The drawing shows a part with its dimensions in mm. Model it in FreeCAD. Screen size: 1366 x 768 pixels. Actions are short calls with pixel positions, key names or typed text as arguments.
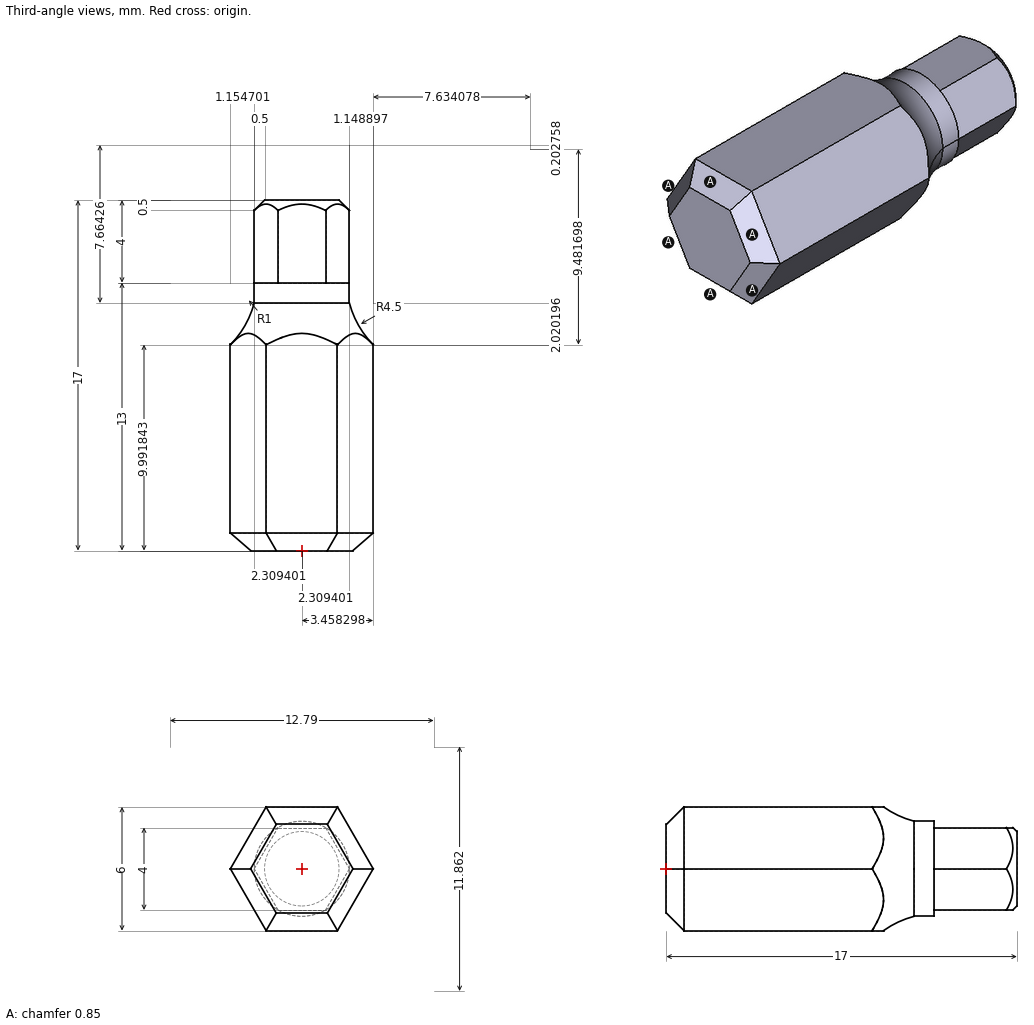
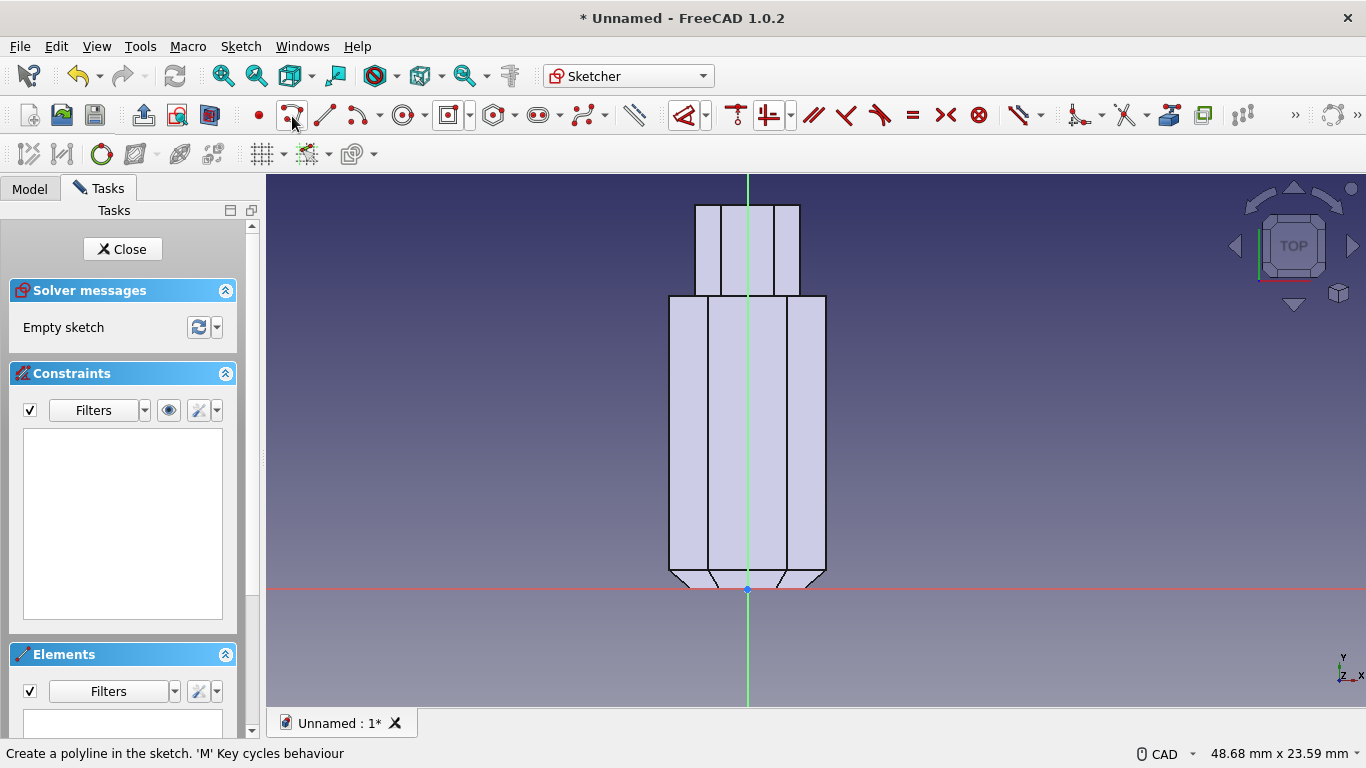
click(695, 296)
click(669, 296)
click(669, 318)
right_click(669, 318)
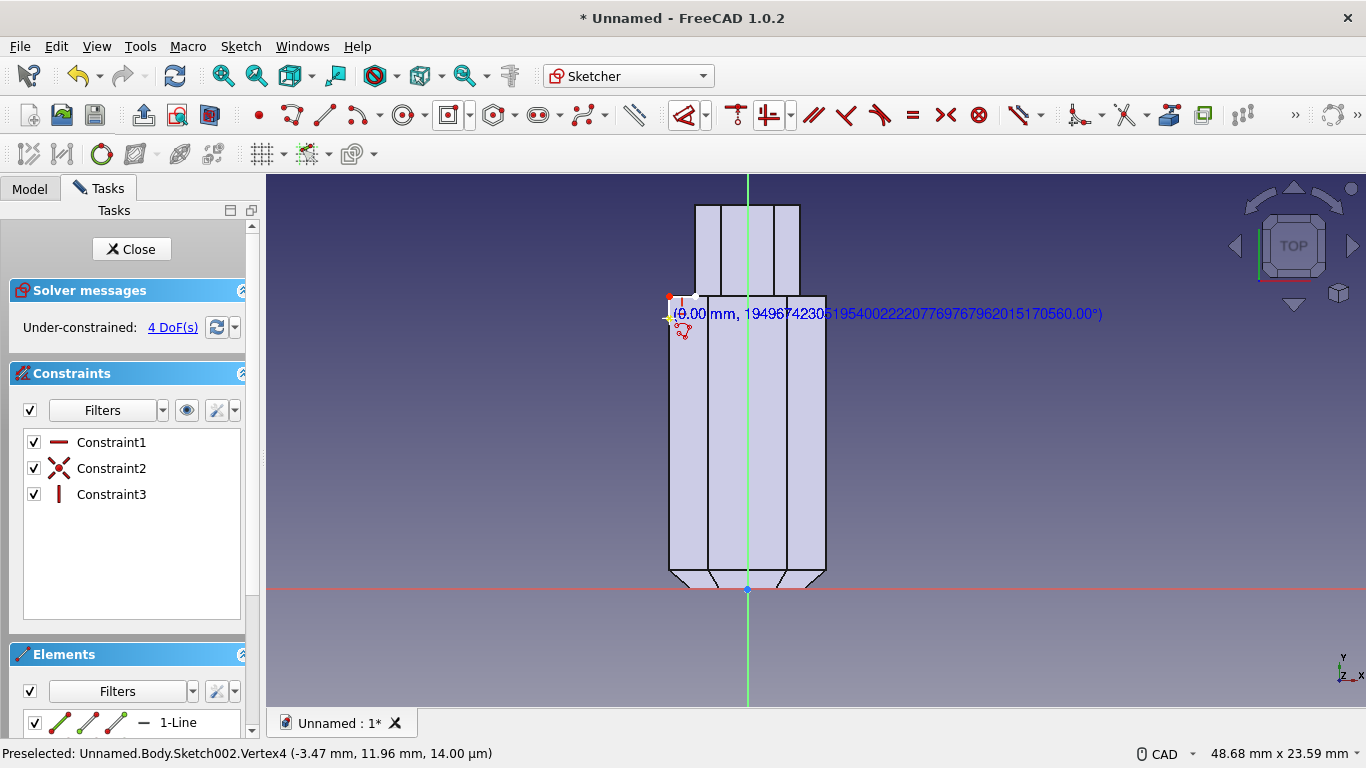
click(380, 116)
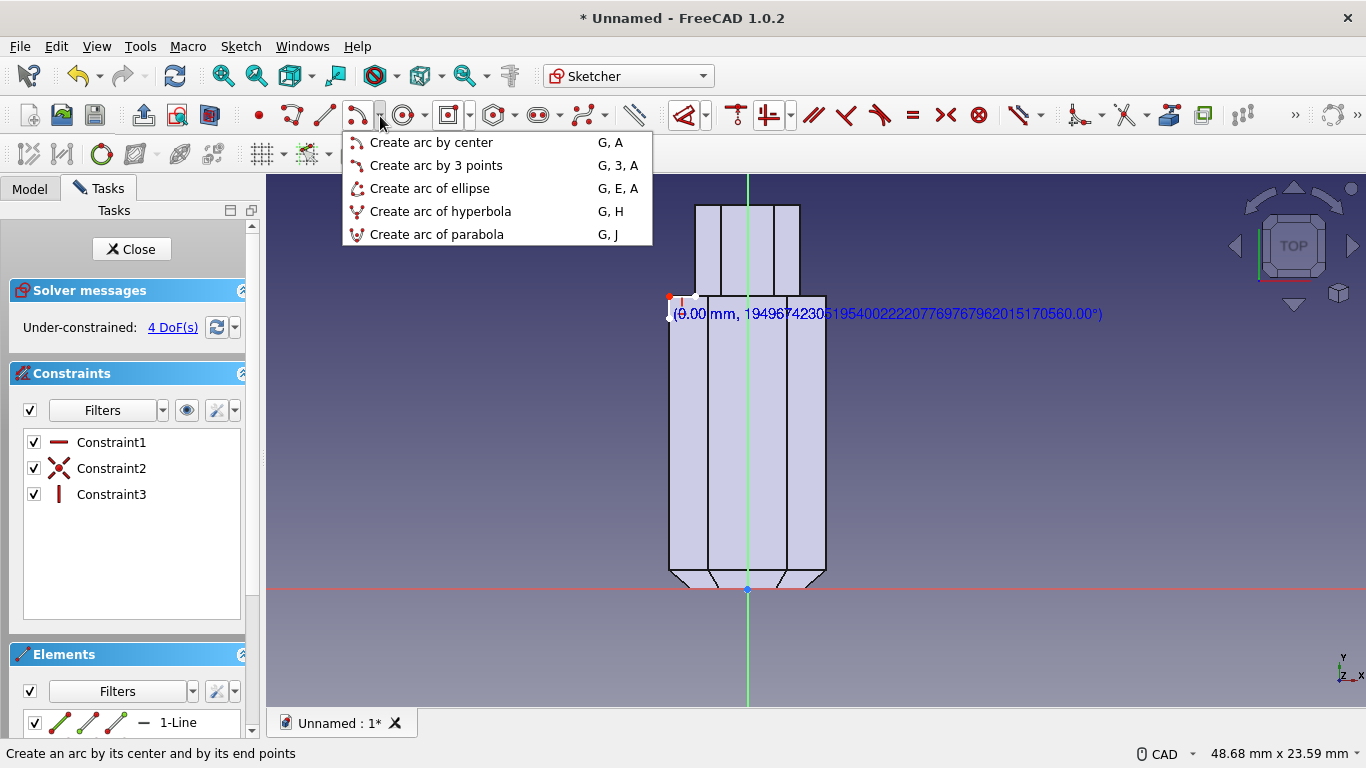
click(498, 166)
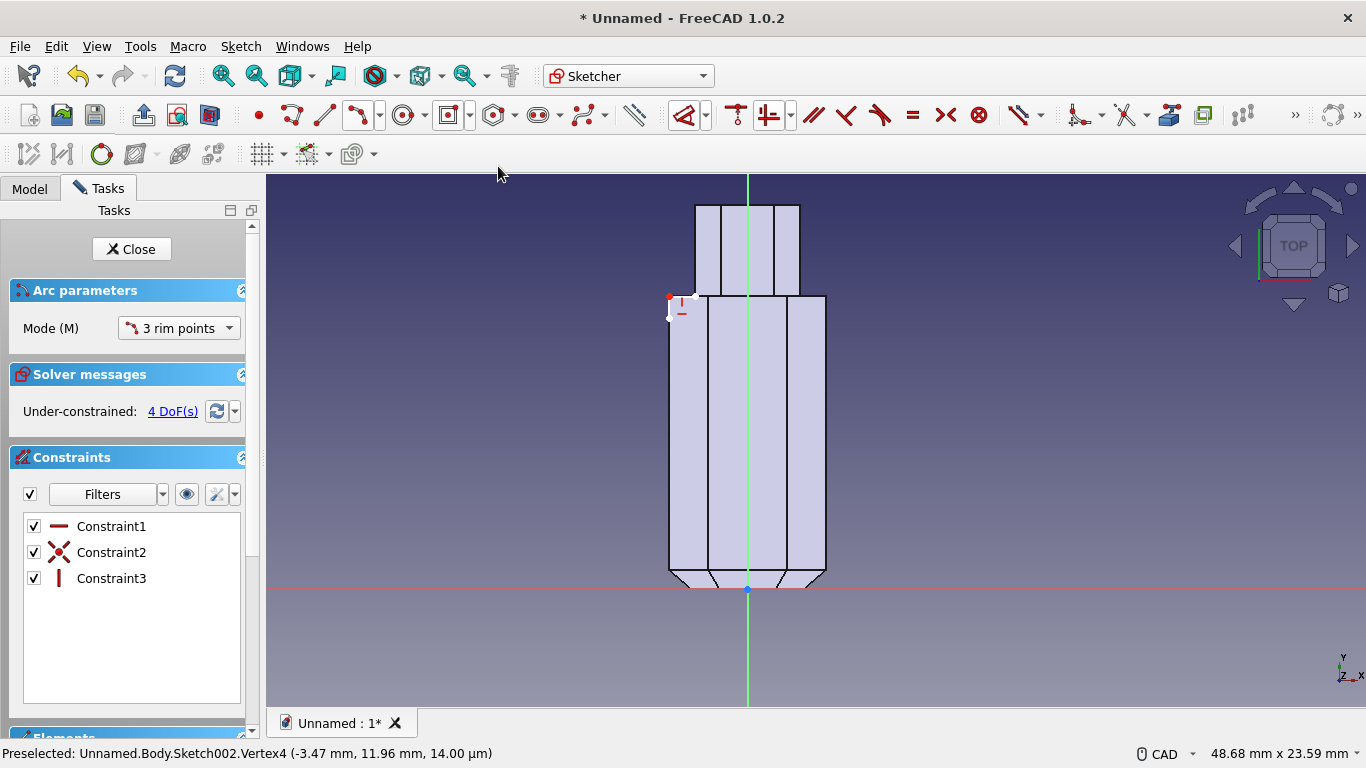
scroll(669, 318, up, 2)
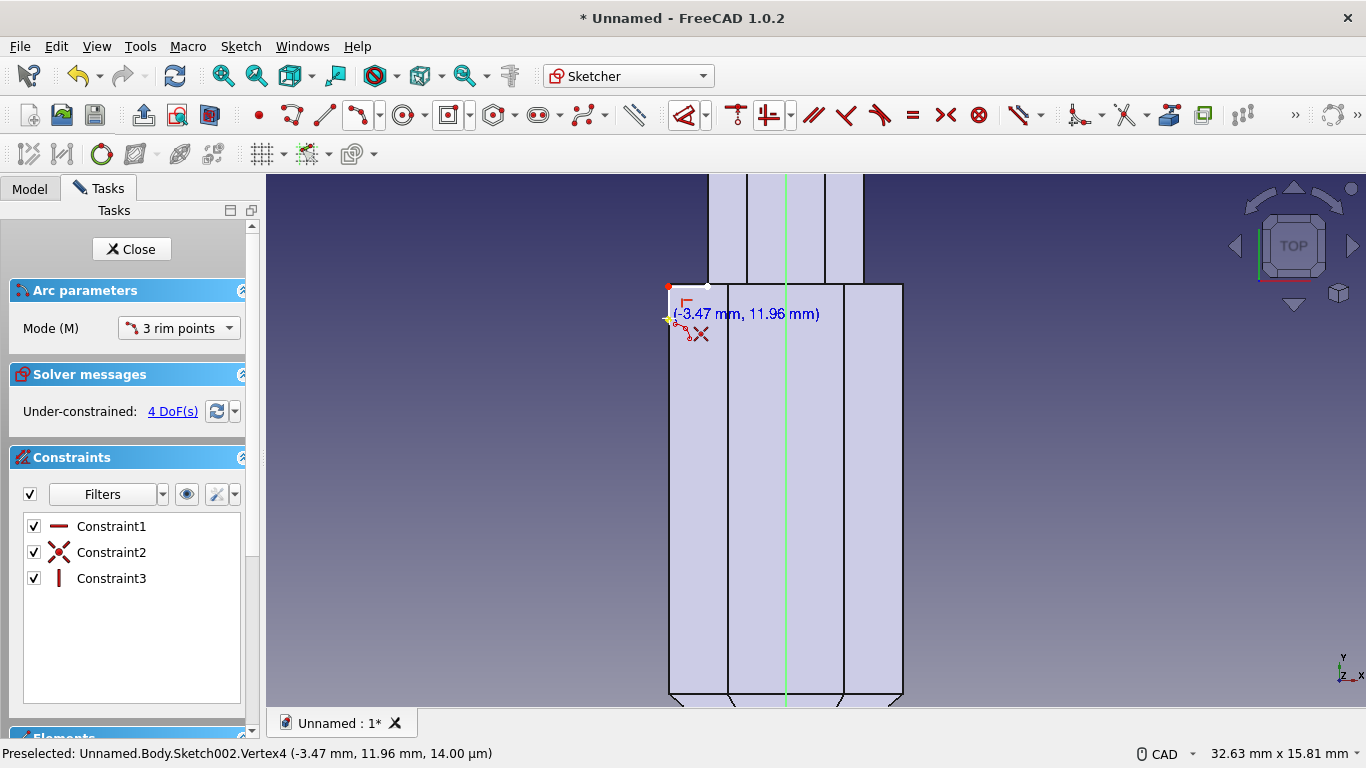
click(669, 319)
click(708, 287)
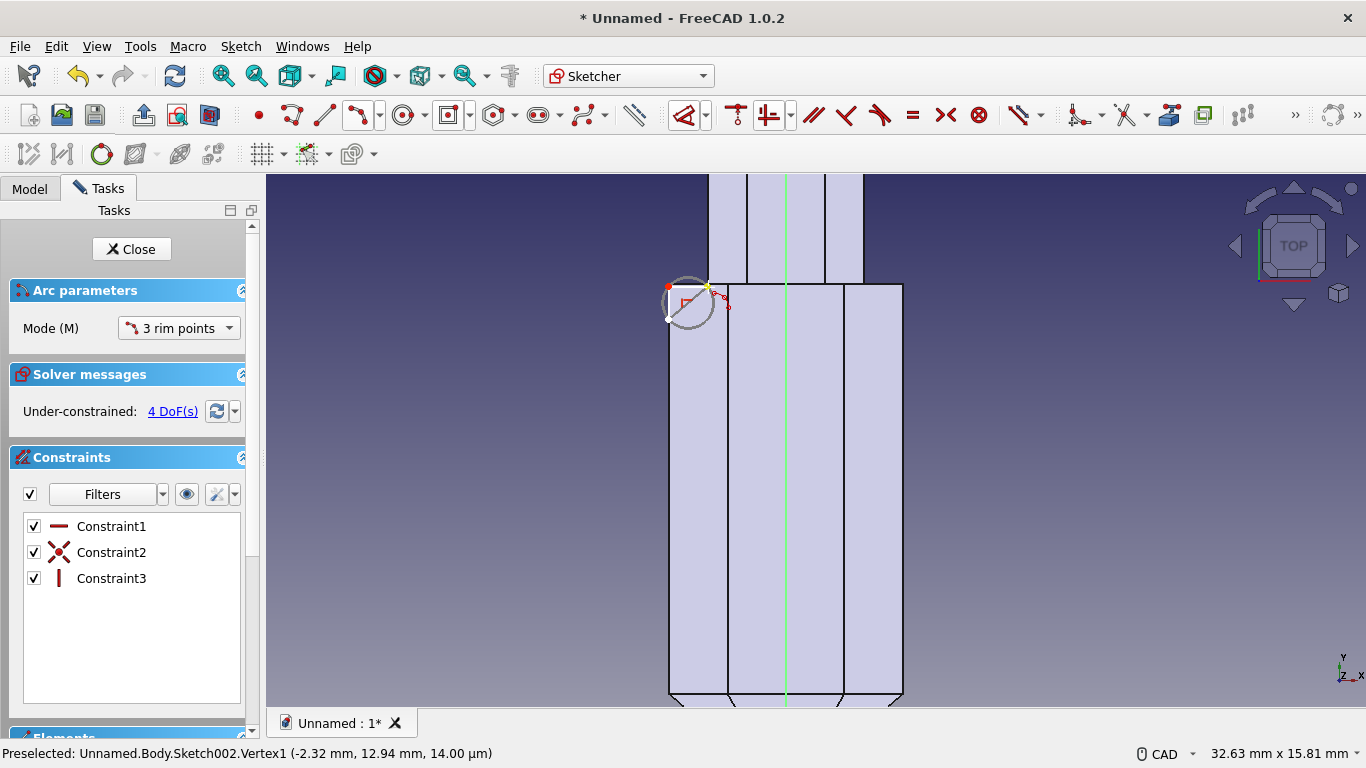
scroll(696, 310, up, 2)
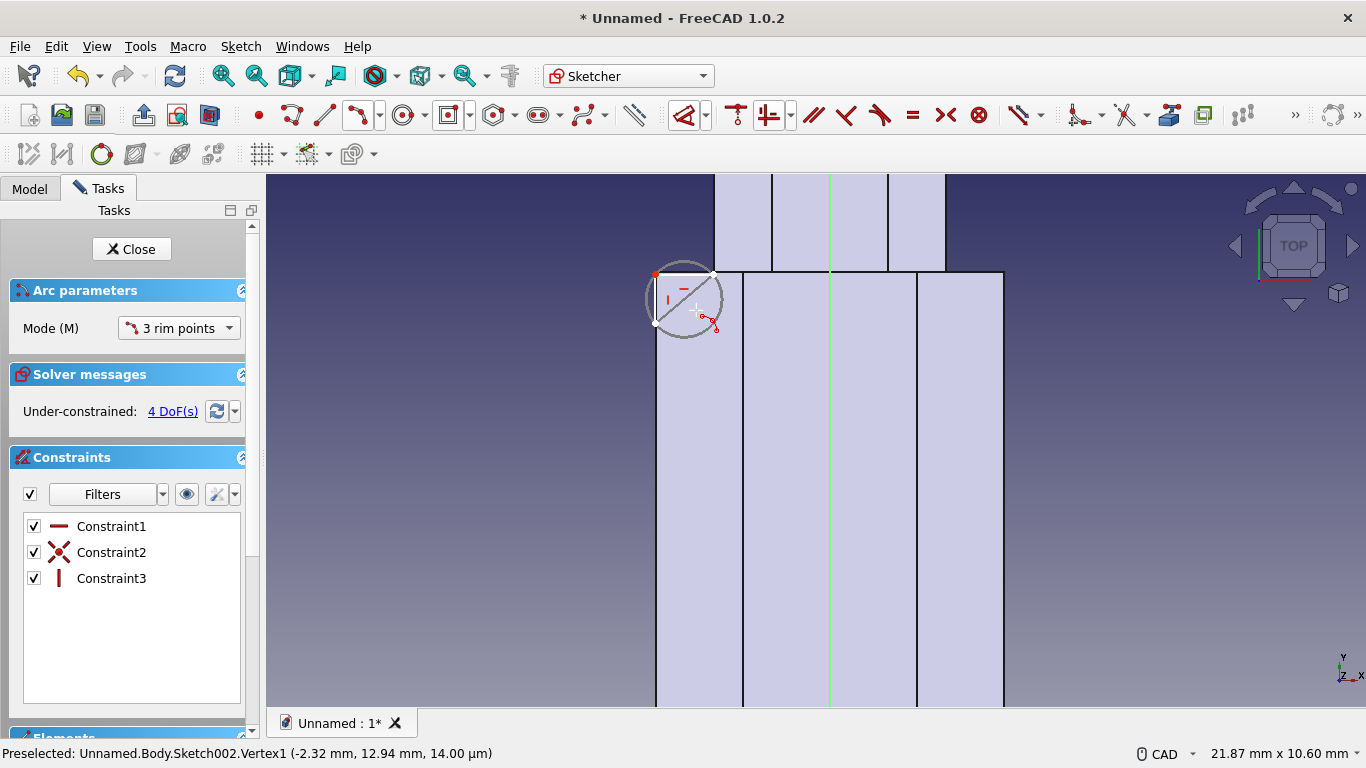
click(696, 310)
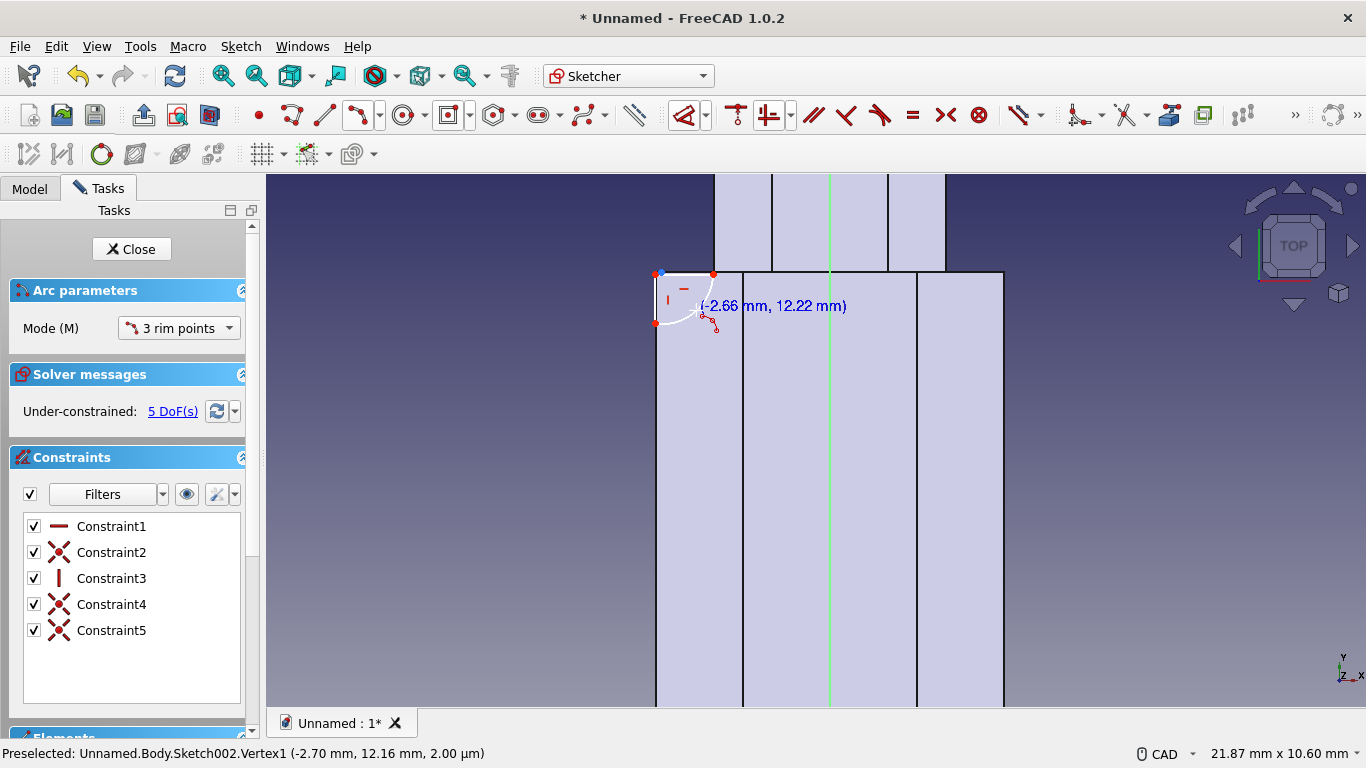
click(292, 116)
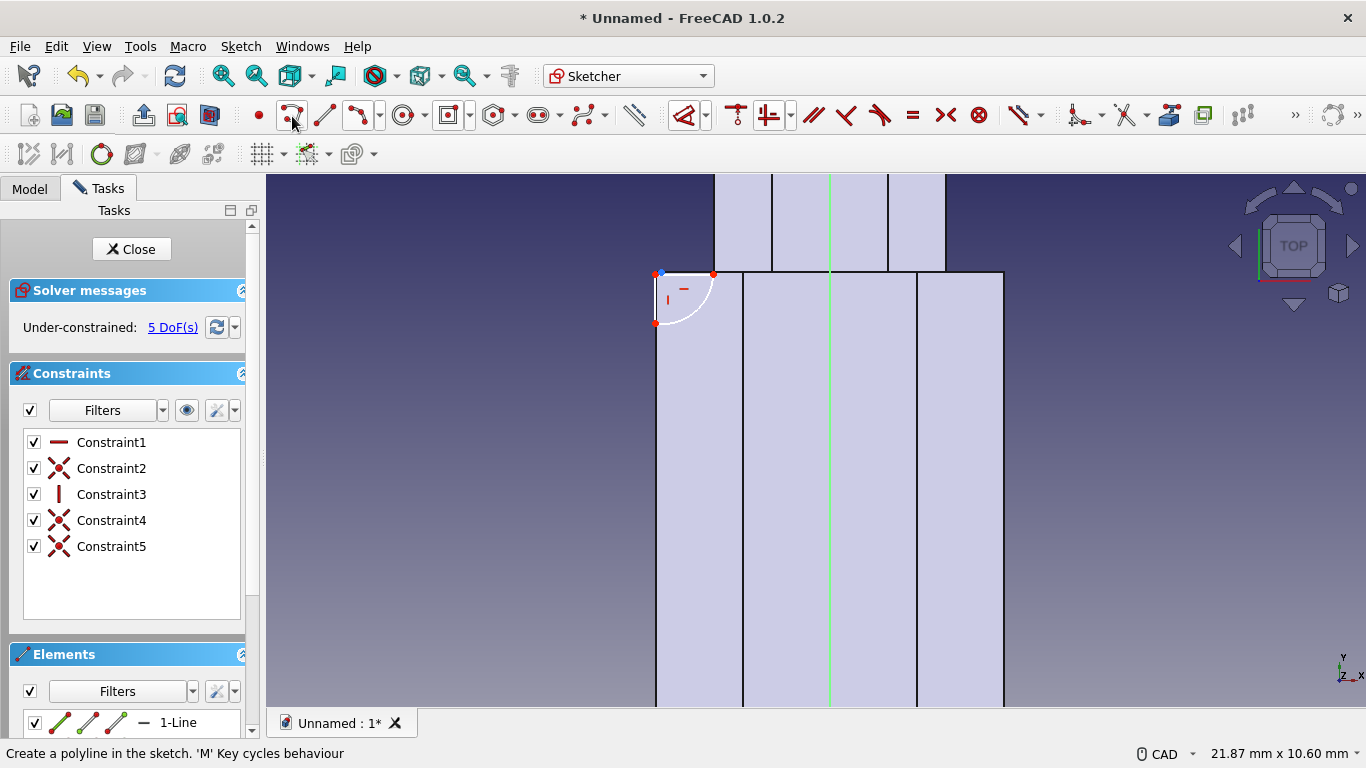
click(1004, 423)
click(1004, 321)
click(946, 321)
right_click(946, 321)